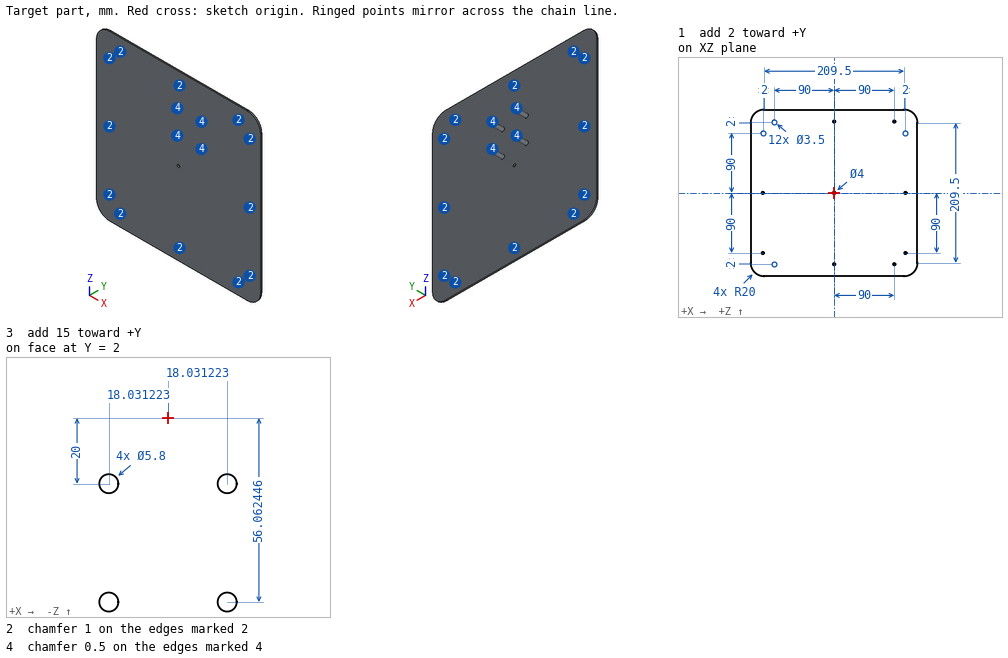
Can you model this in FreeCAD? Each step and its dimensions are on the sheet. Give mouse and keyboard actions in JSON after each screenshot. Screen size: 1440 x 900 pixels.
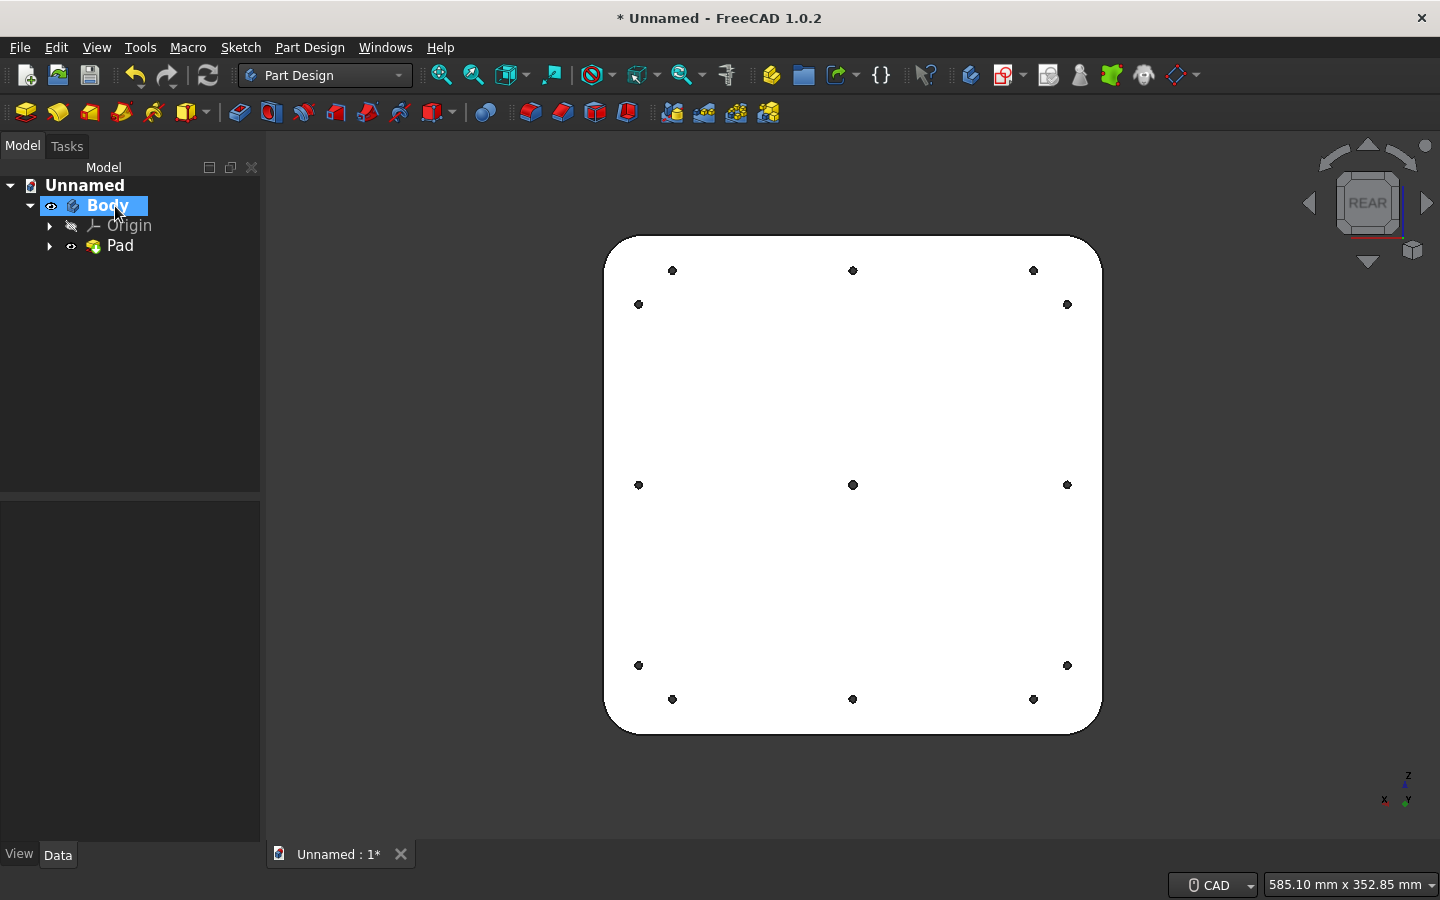
{"action": "left_click", "coordinate": [1037, 698]}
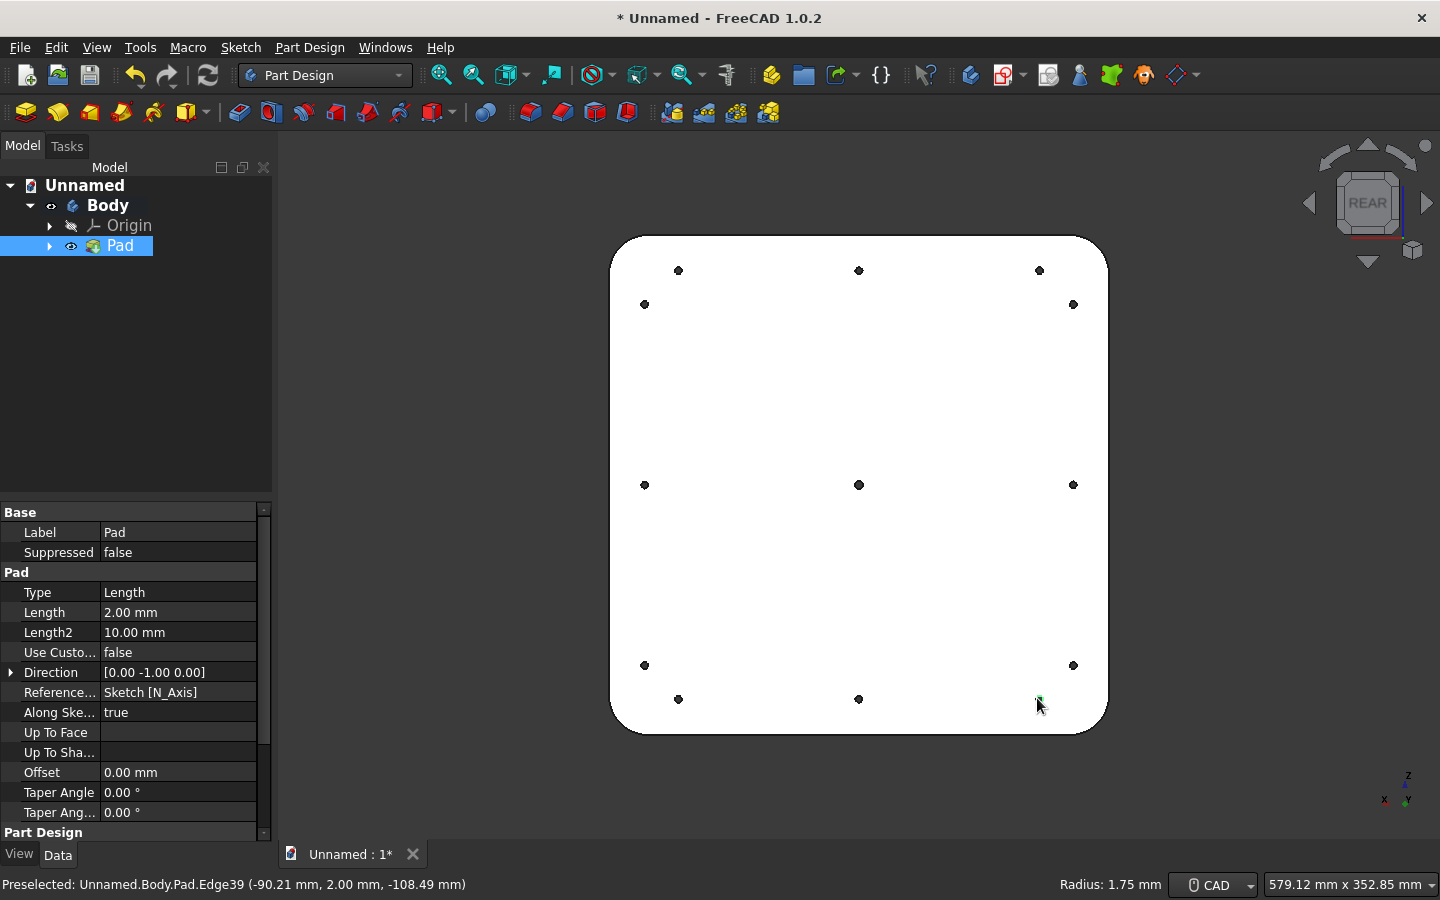
{"action": "left_click", "coordinate": [863, 698], "text": "ctrl"}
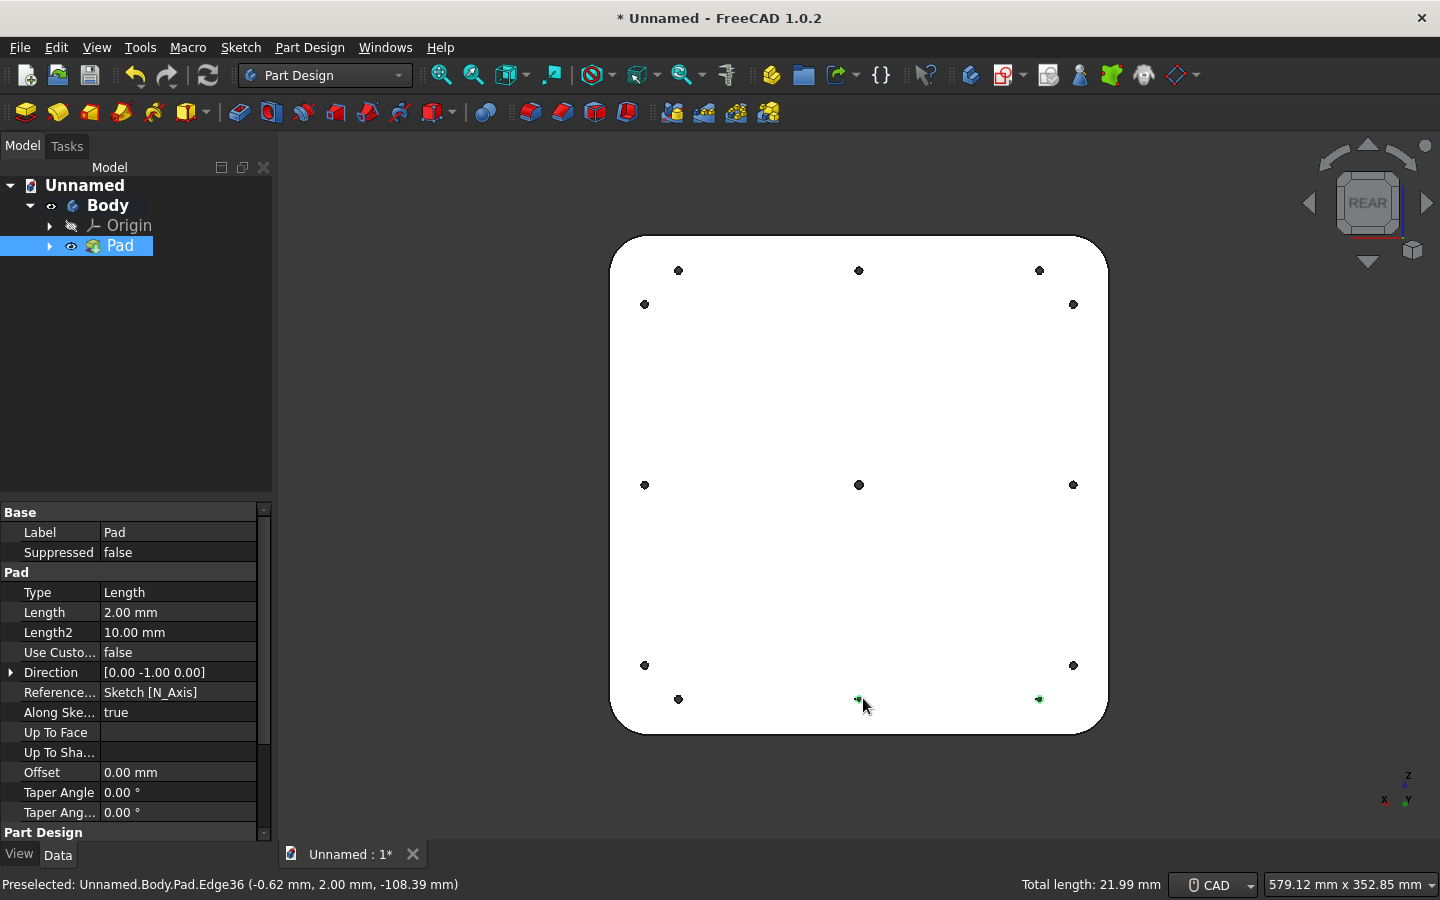
{"action": "left_click", "coordinate": [682, 698], "text": "ctrl"}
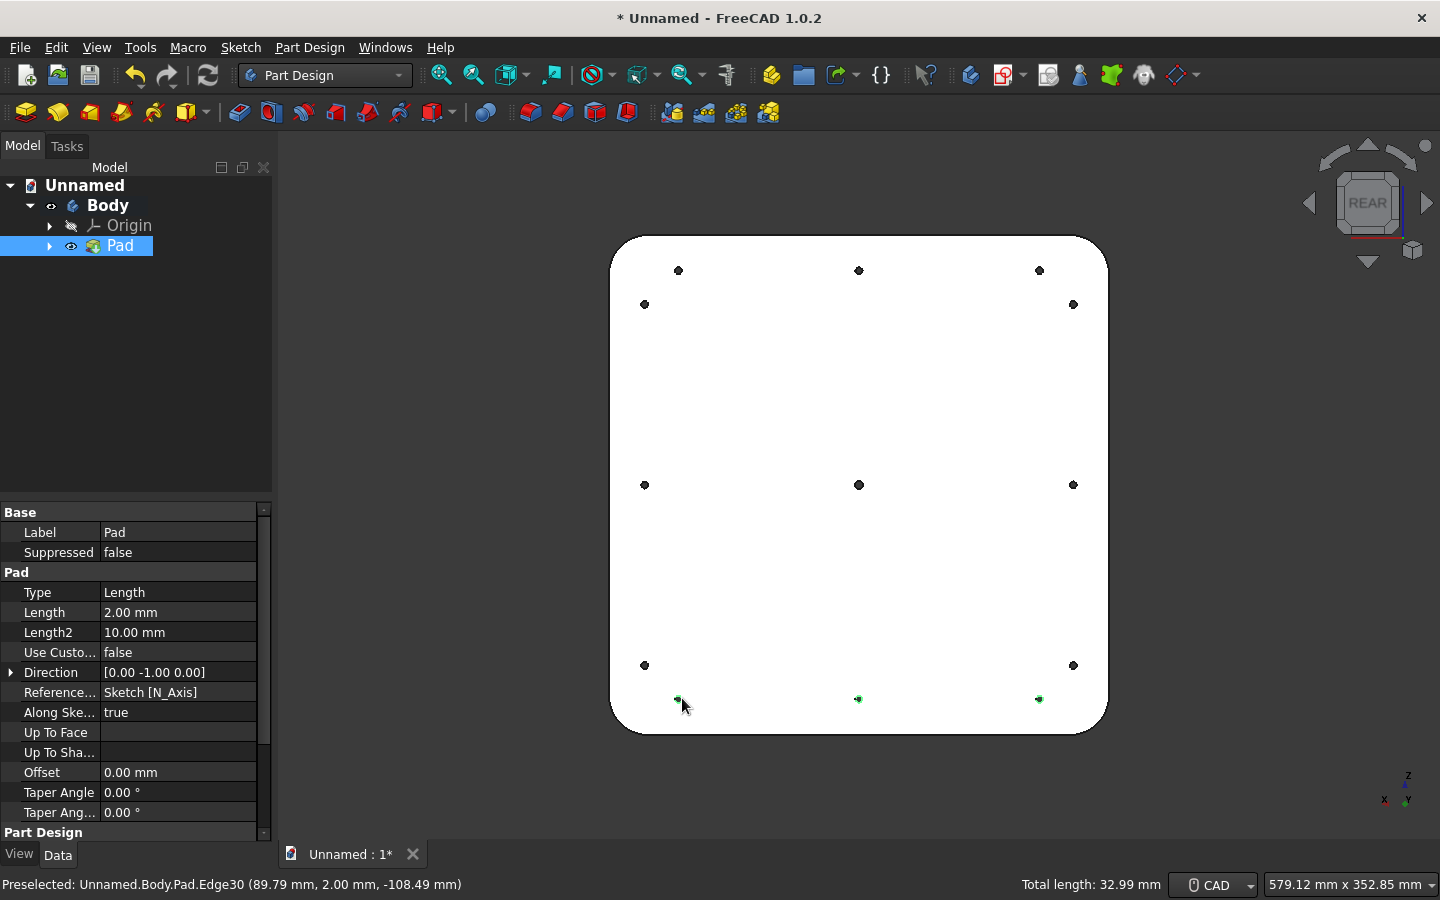
{"action": "left_click", "coordinate": [648, 665], "text": "ctrl"}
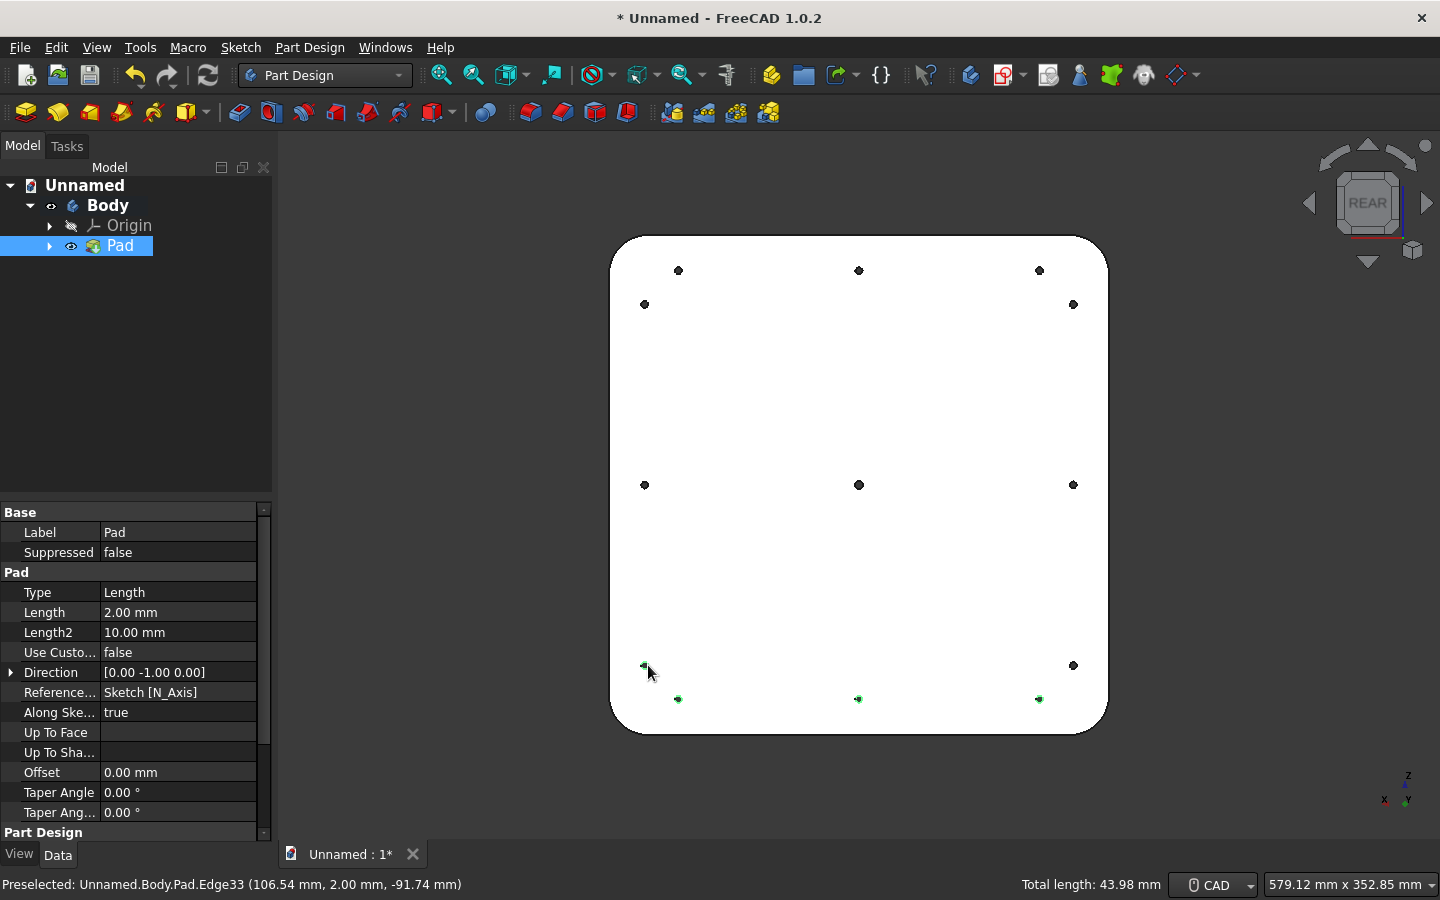
{"action": "left_click", "coordinate": [648, 484], "text": "ctrl"}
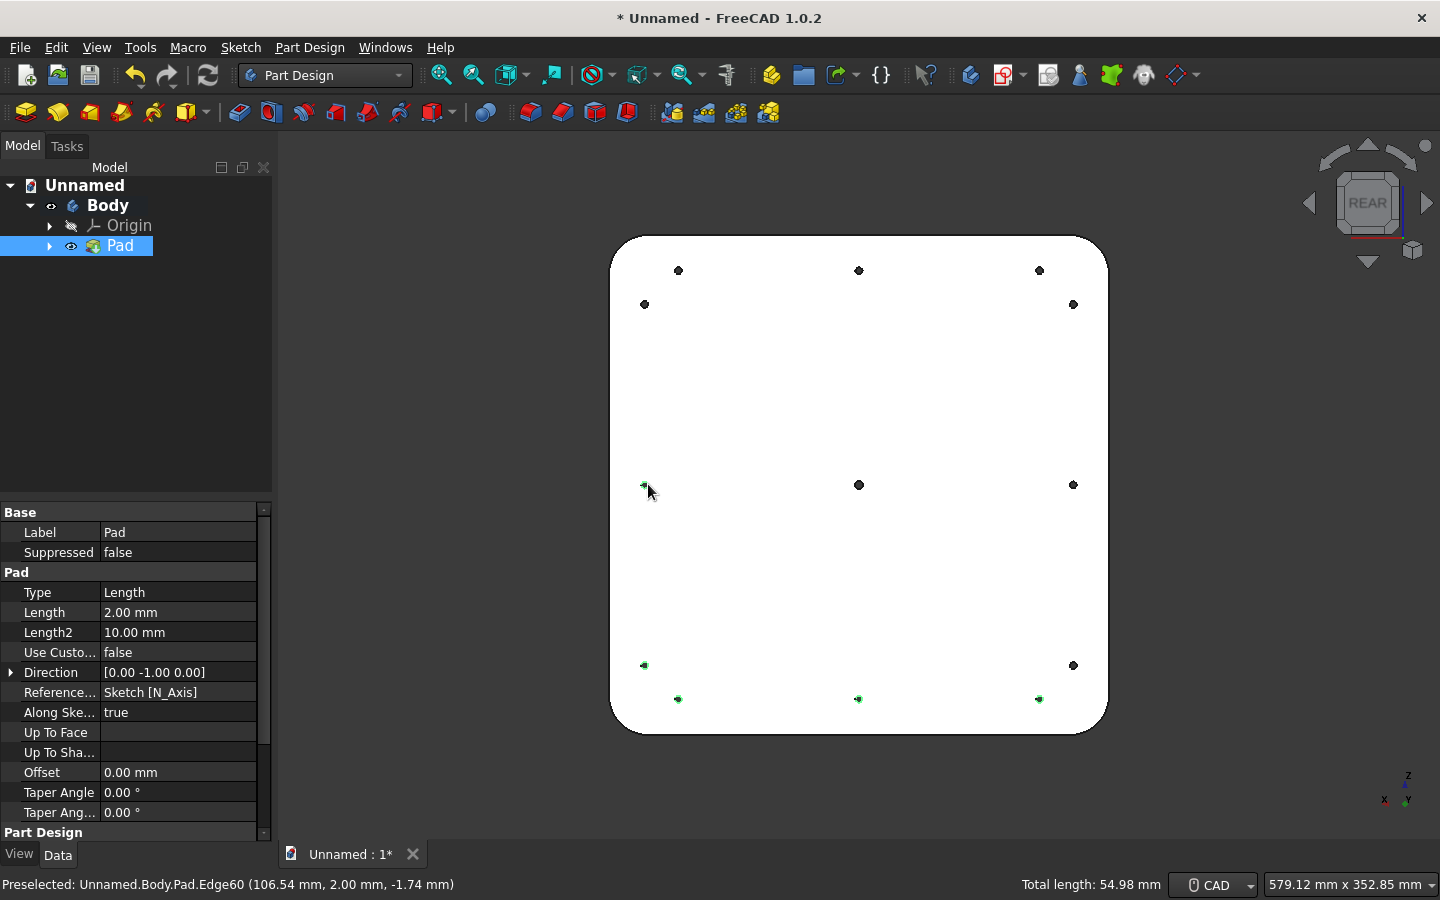
{"action": "left_click", "coordinate": [648, 303], "text": "ctrl"}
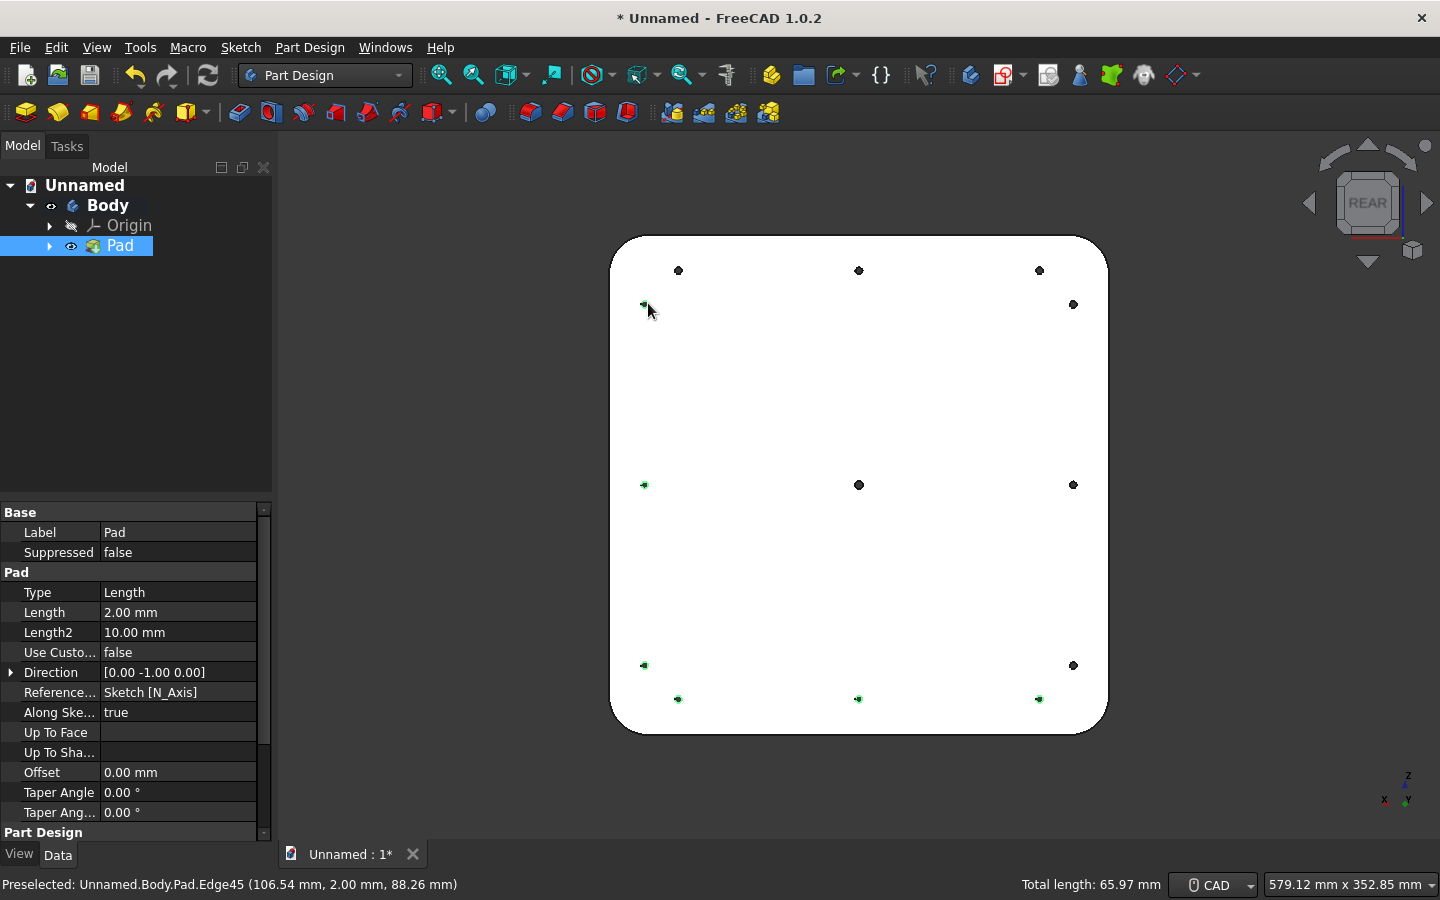
{"action": "left_click", "coordinate": [682, 270], "text": "ctrl"}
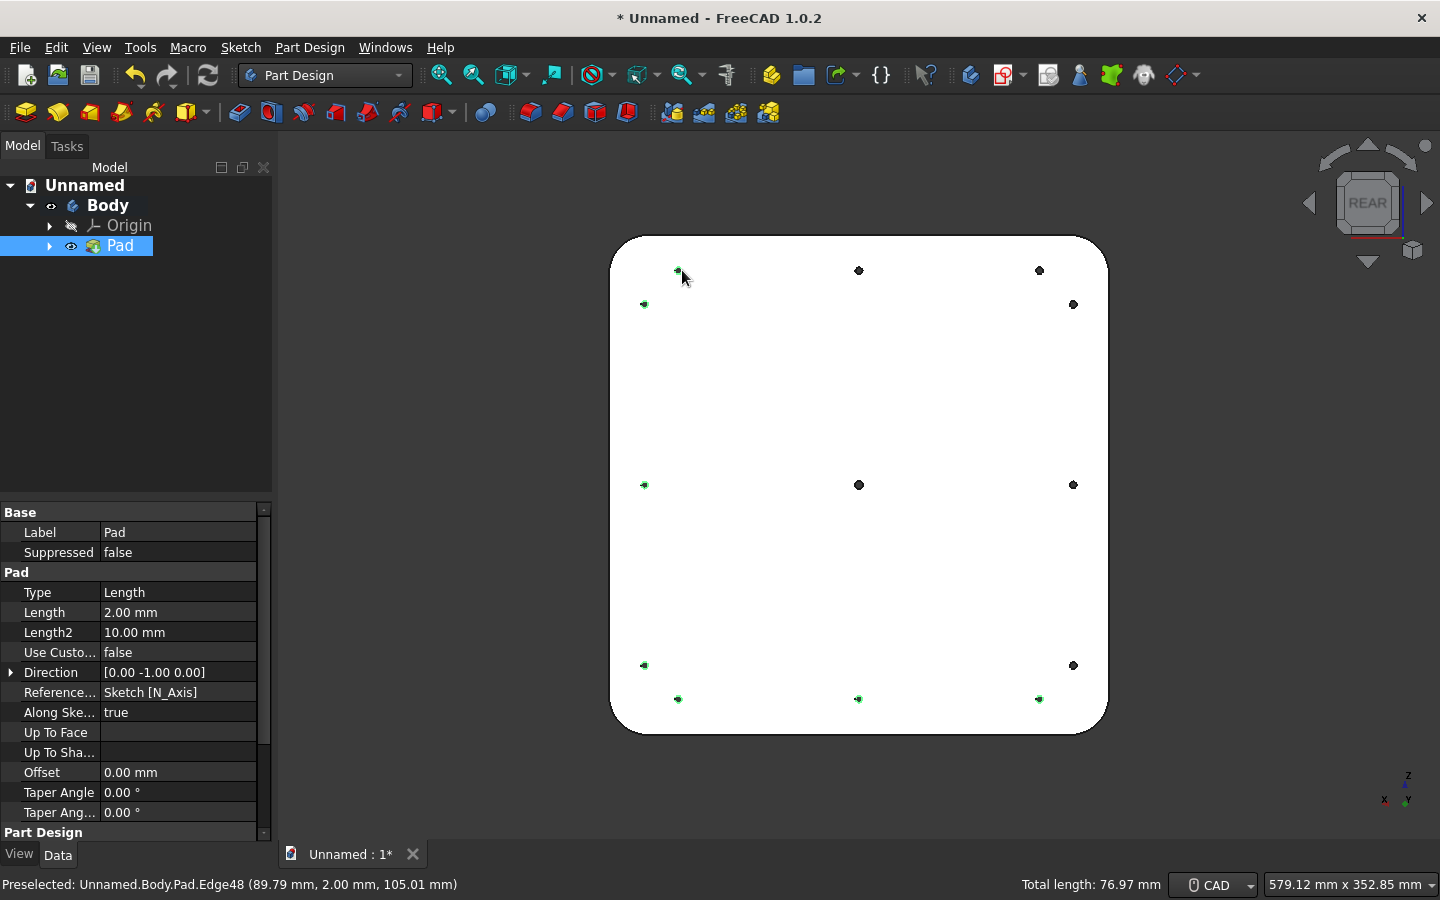
{"action": "left_click", "coordinate": [863, 270], "text": "ctrl"}